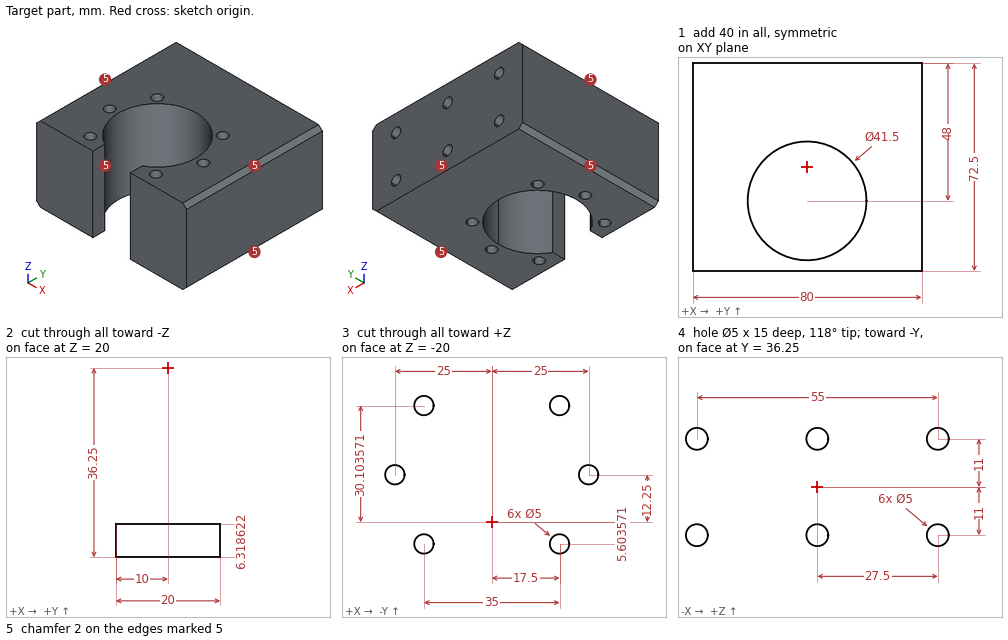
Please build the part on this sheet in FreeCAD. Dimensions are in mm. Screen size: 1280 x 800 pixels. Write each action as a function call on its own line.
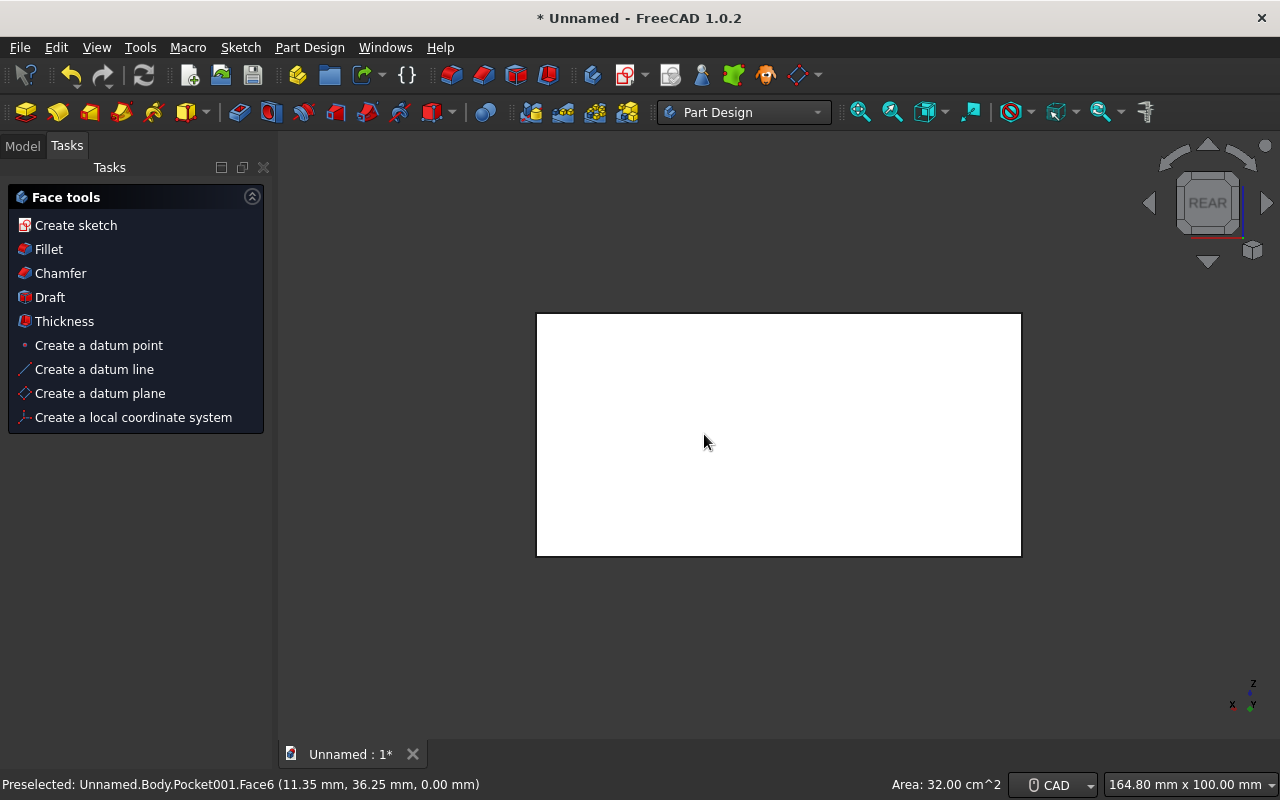
click(626, 76)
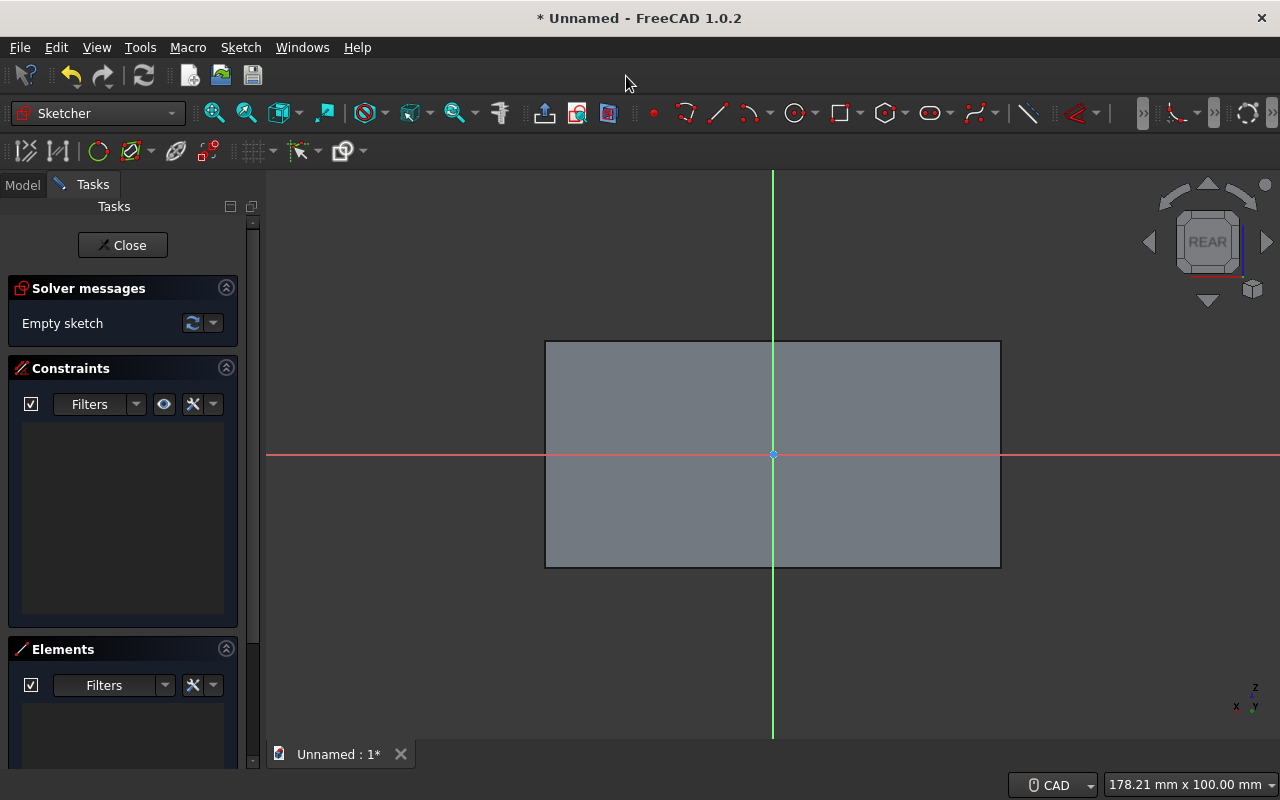
scroll(856, 454, up, 3)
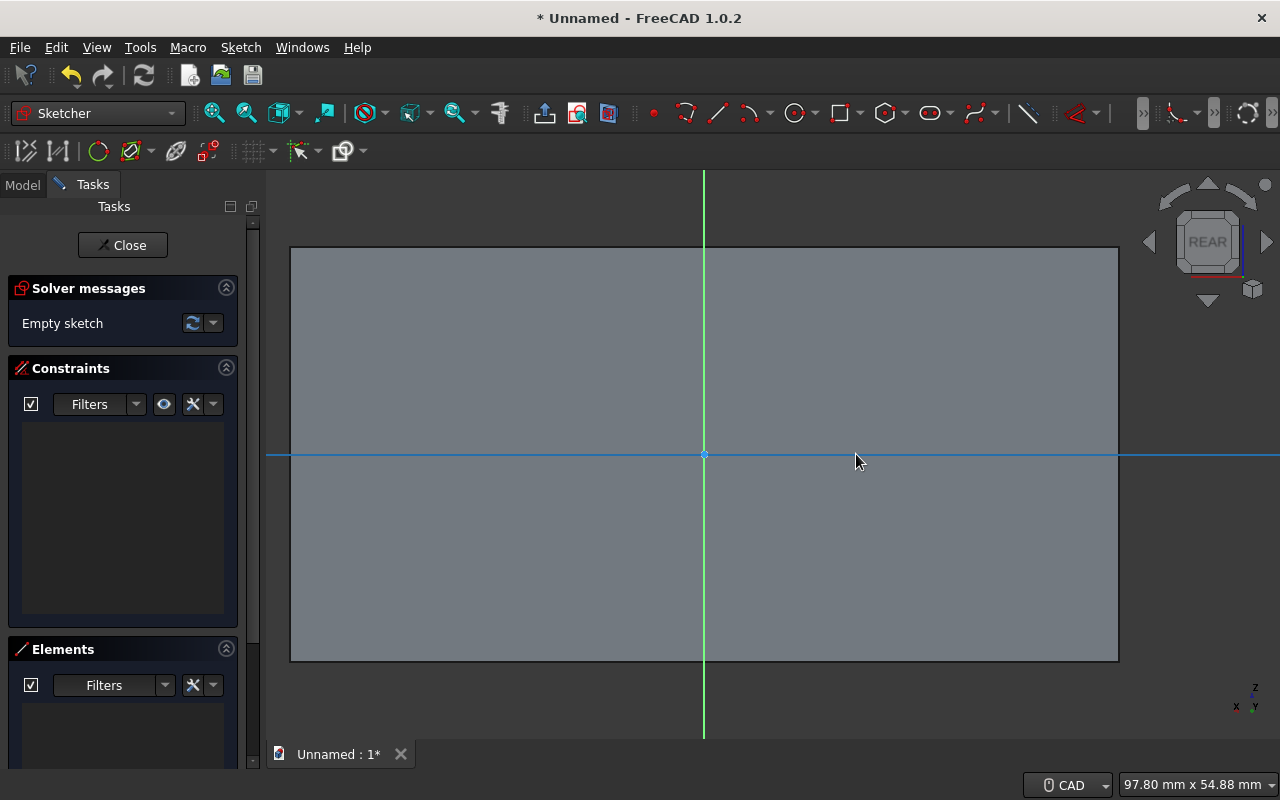
key(g)
key(c)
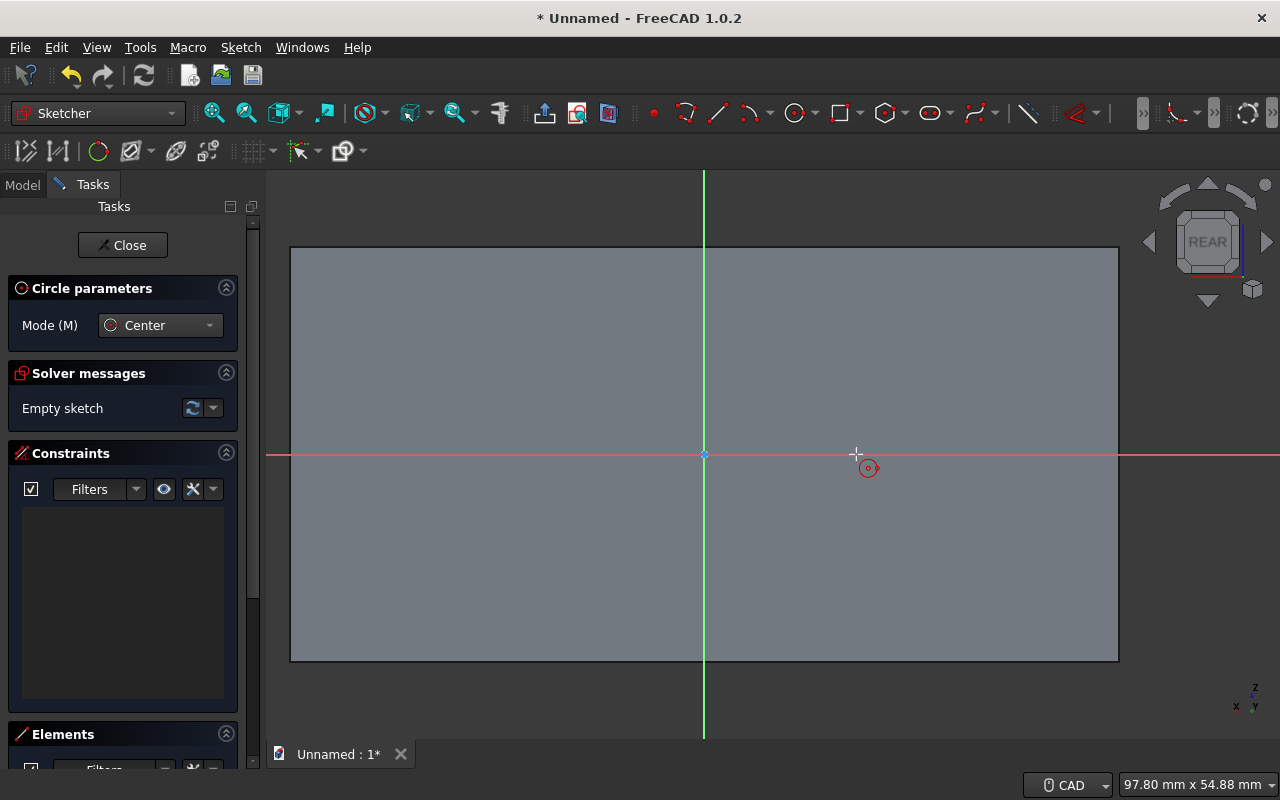
click(989, 569)
move(1008, 550)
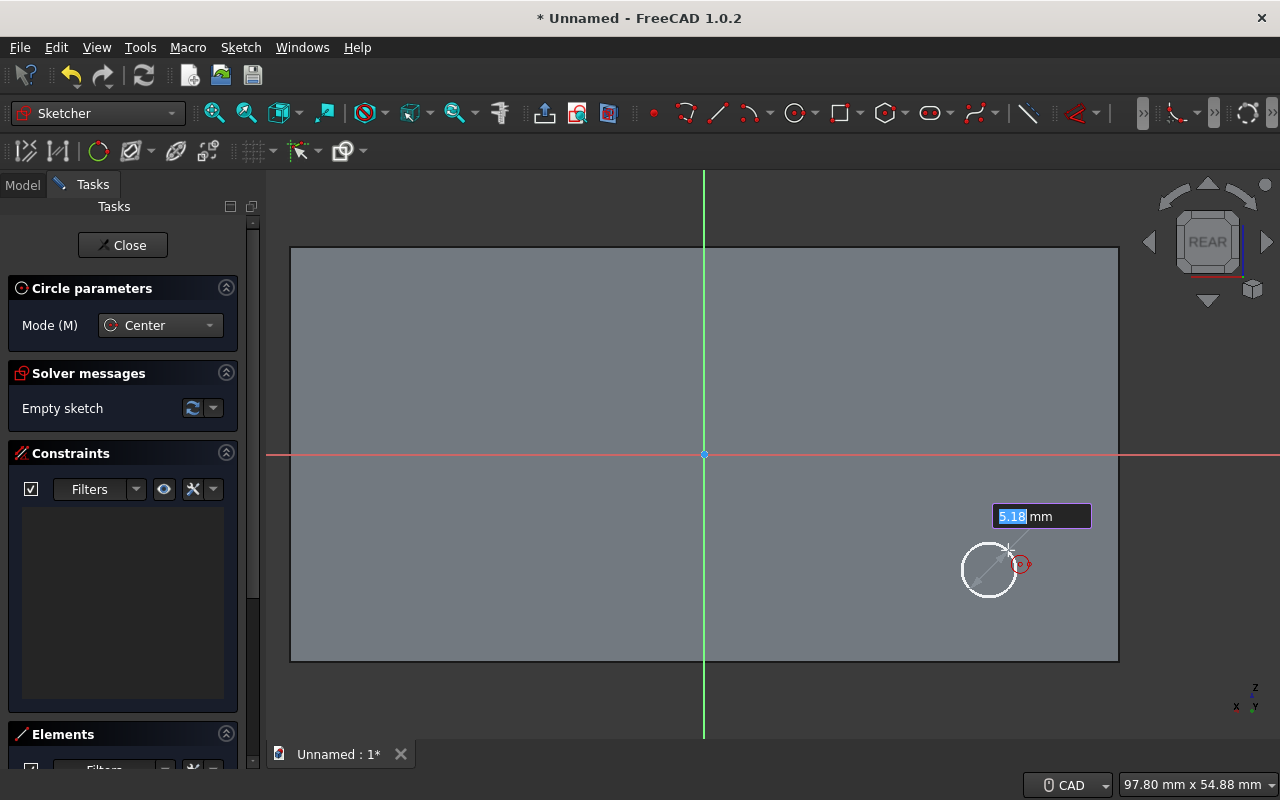
text(5)
key(Return)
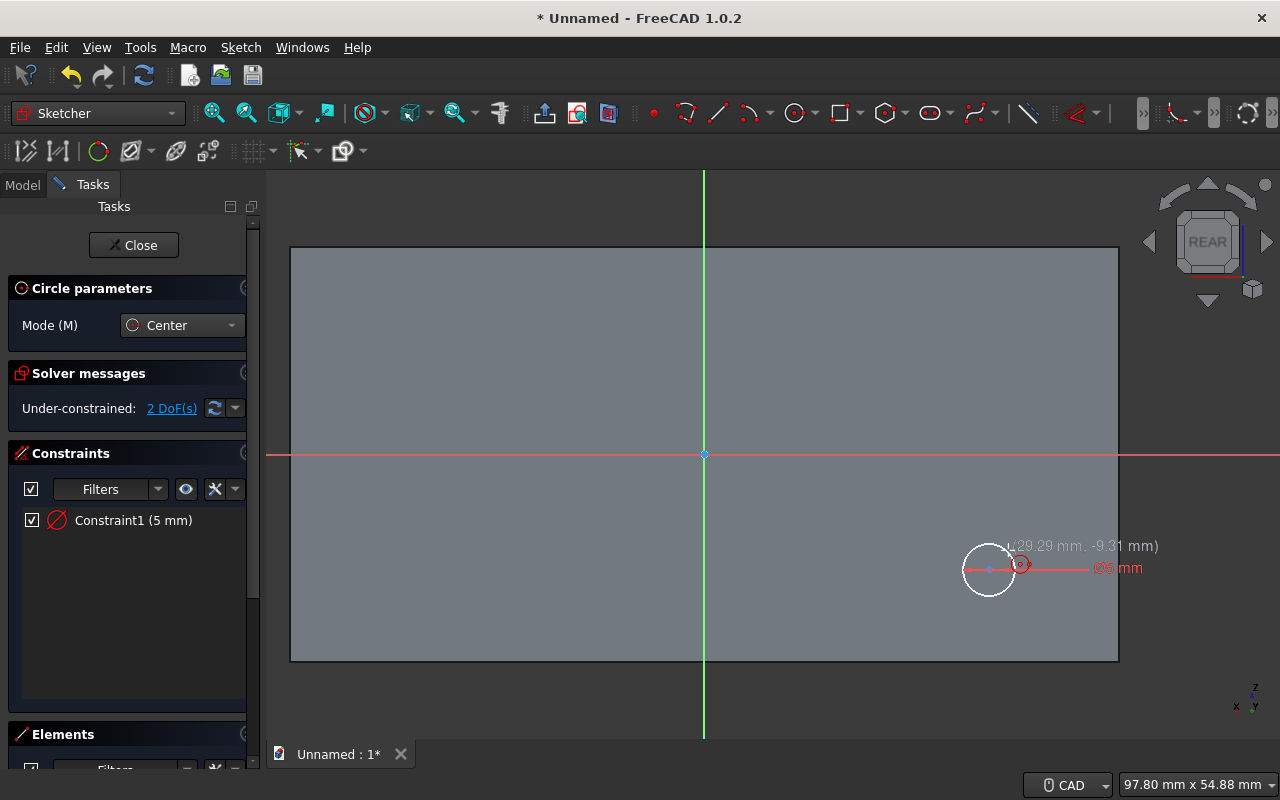
click(989, 340)
move(1008, 322)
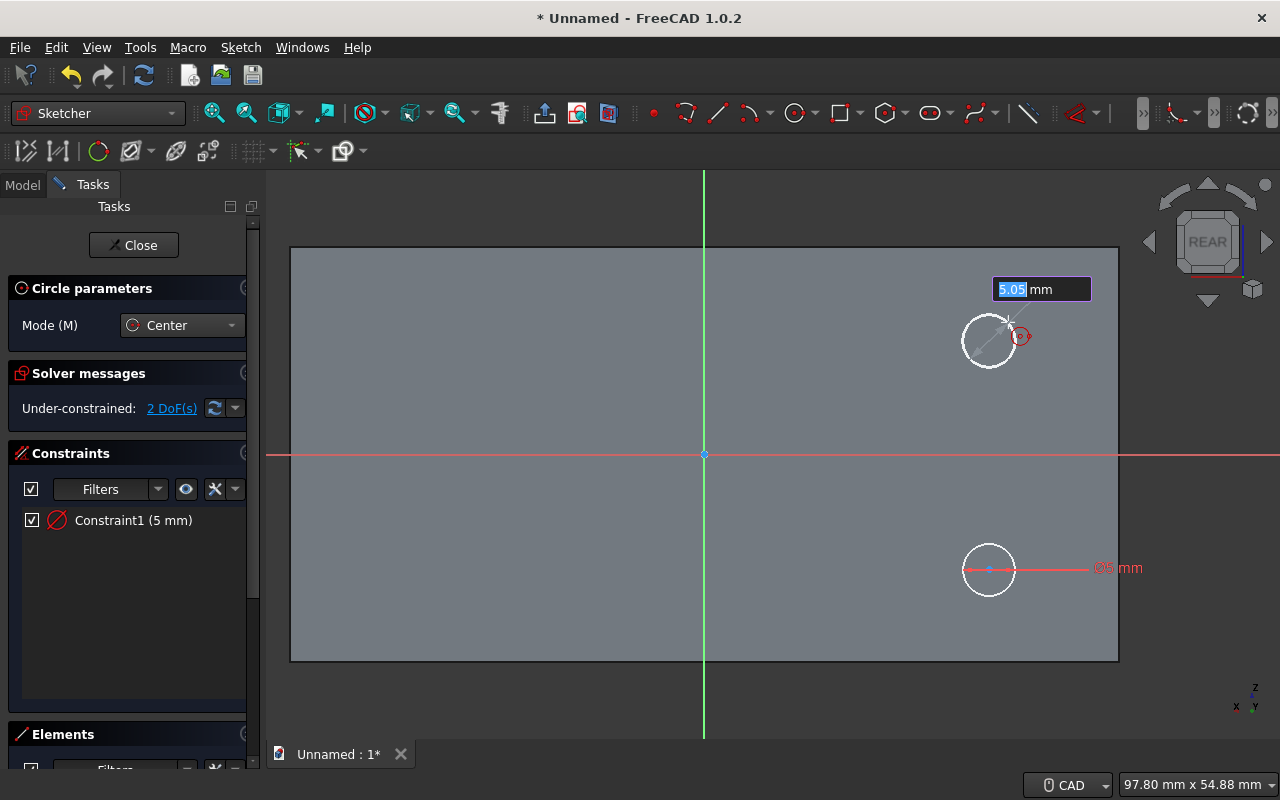
text(5)
key(Return)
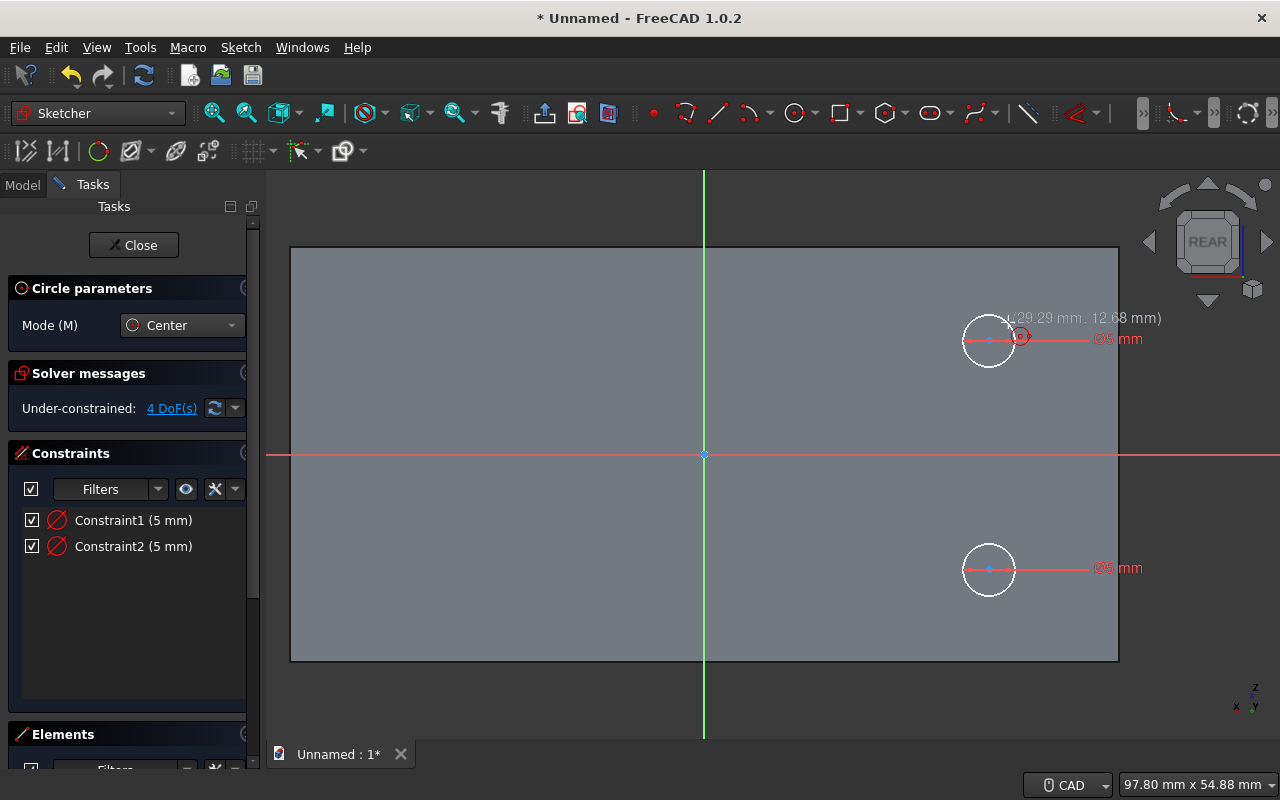
click(419, 340)
move(437, 322)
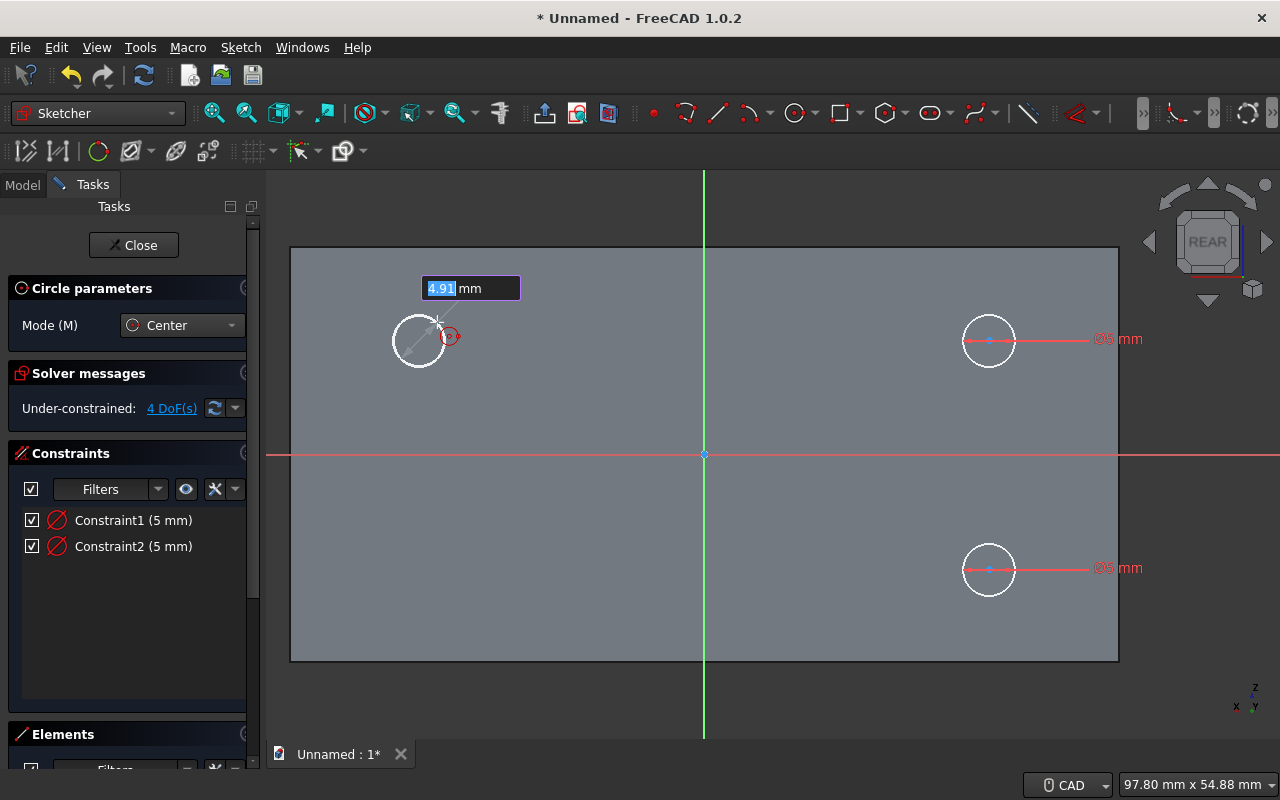
text(5)
key(Return)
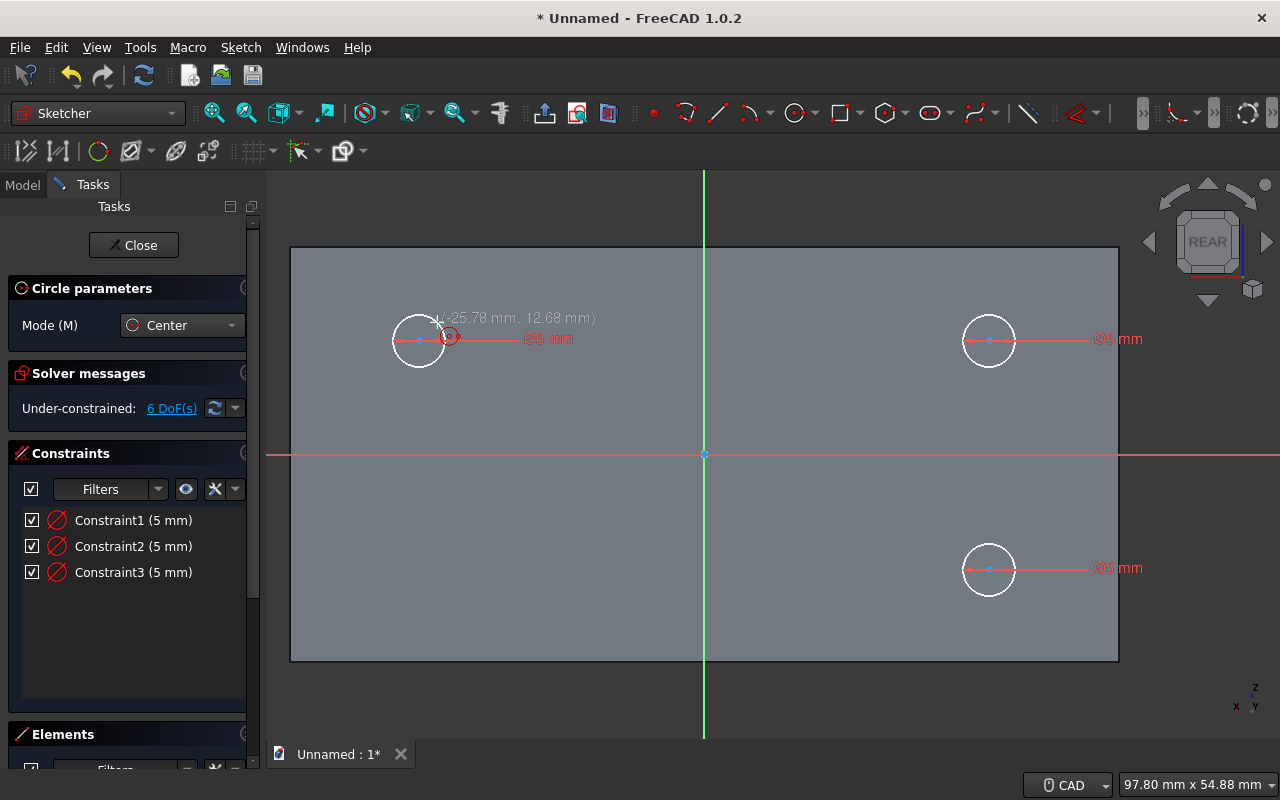
click(419, 569)
move(437, 550)